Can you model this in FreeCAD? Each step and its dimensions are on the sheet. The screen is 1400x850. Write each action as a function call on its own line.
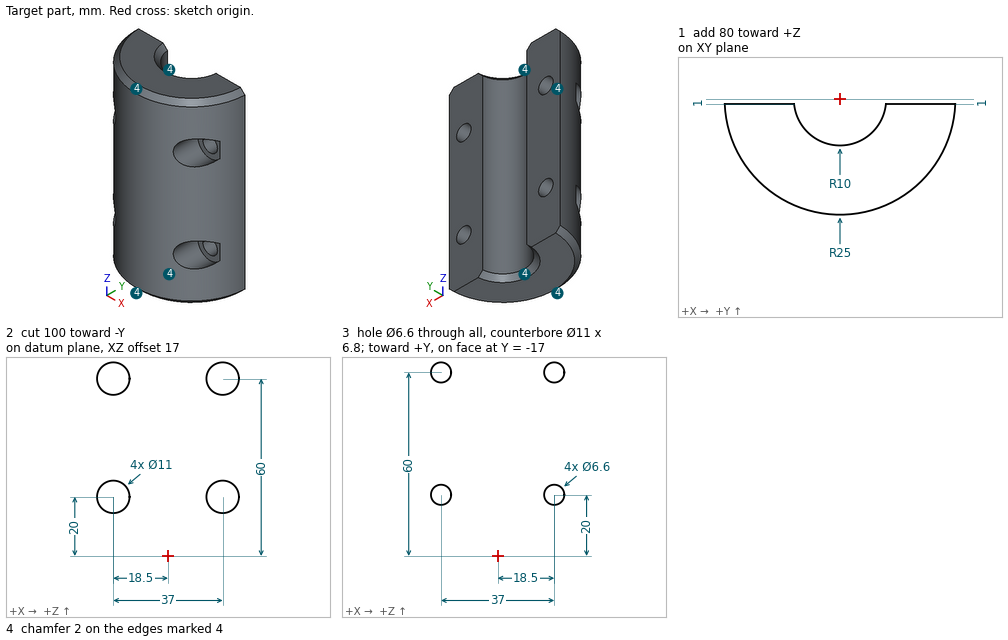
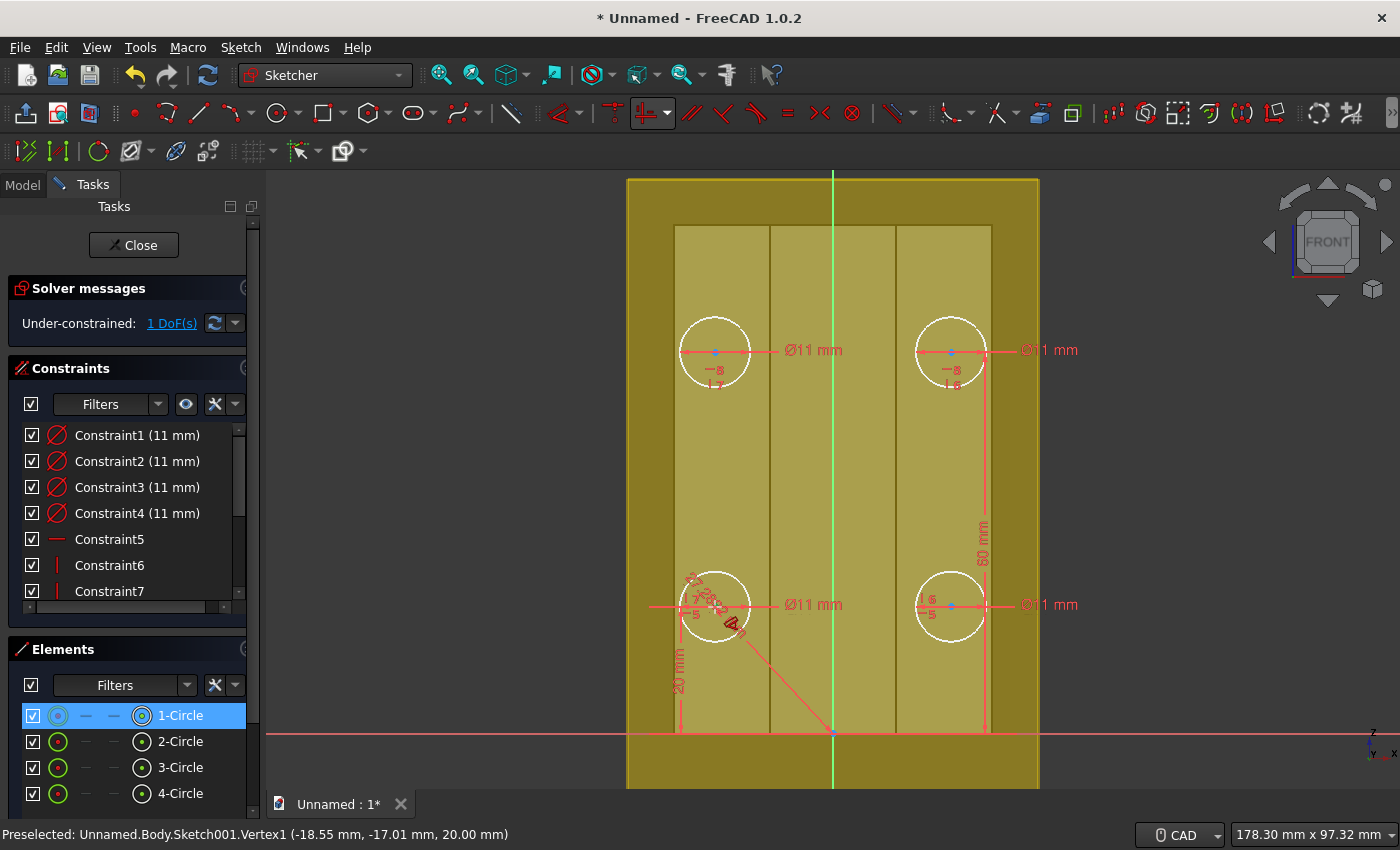
click(951, 607)
click(779, 641)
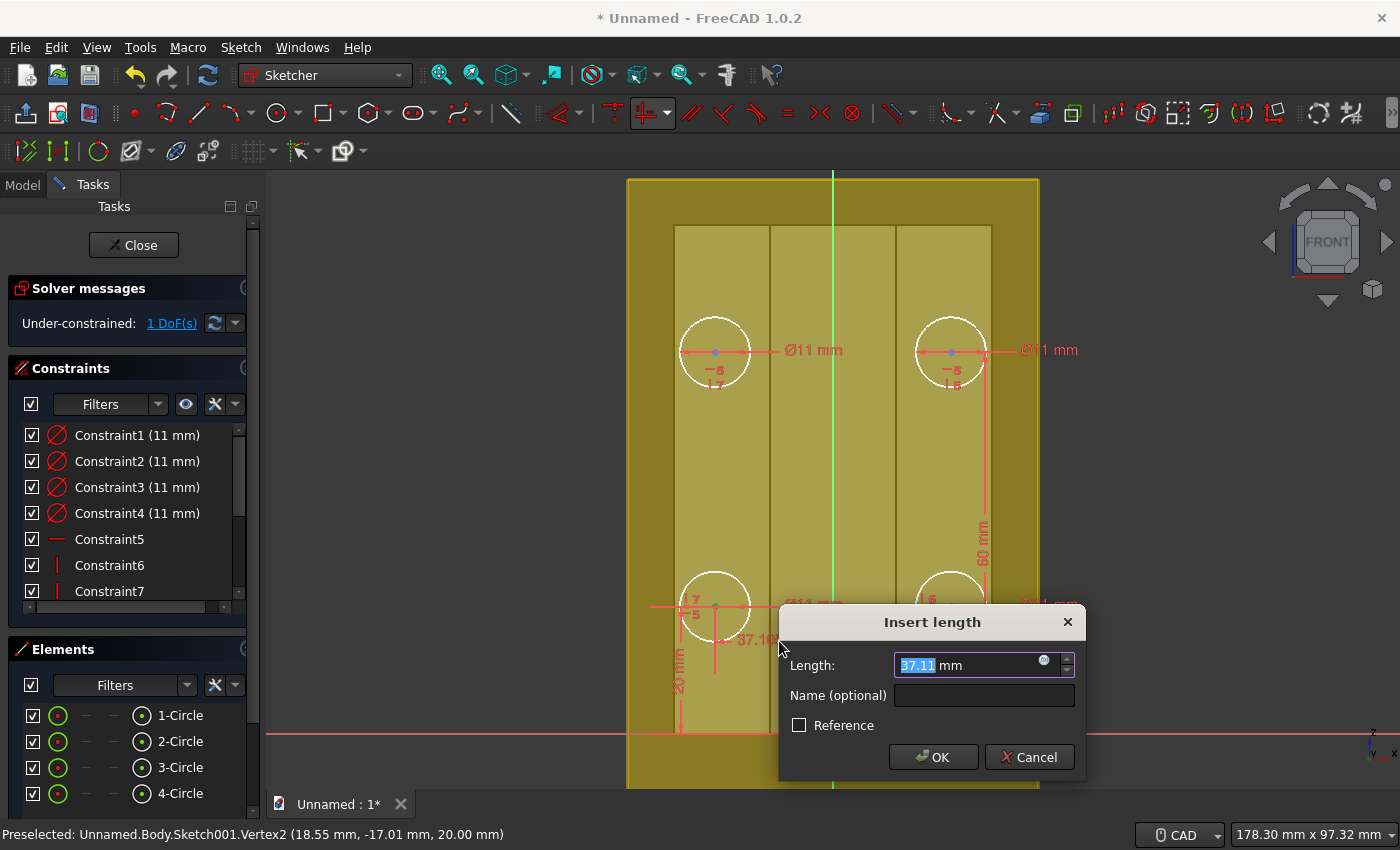
text(37)
key(Return)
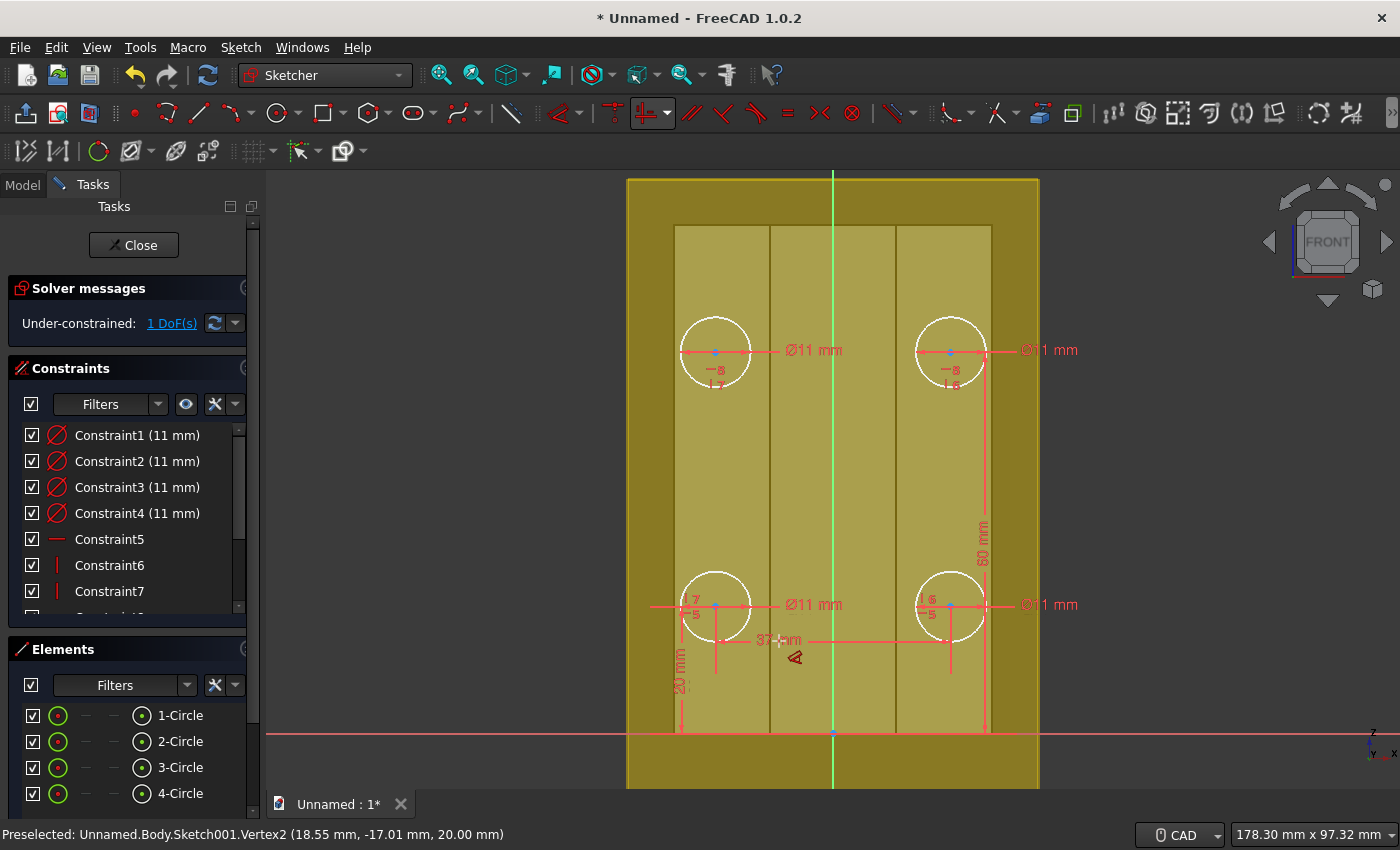
click(716, 607)
click(774, 573)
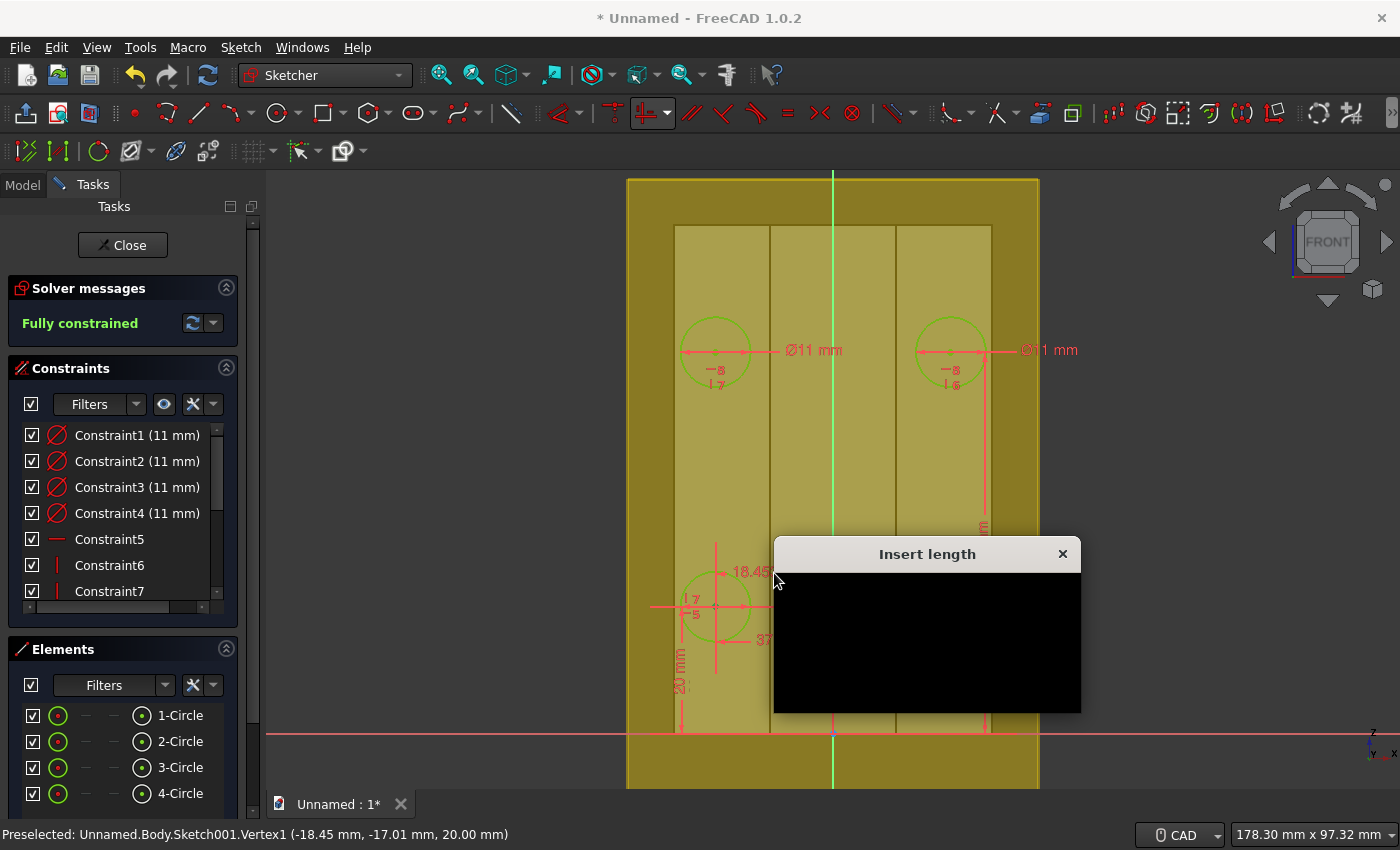
text(18.5)
key(Return)
key(Escape)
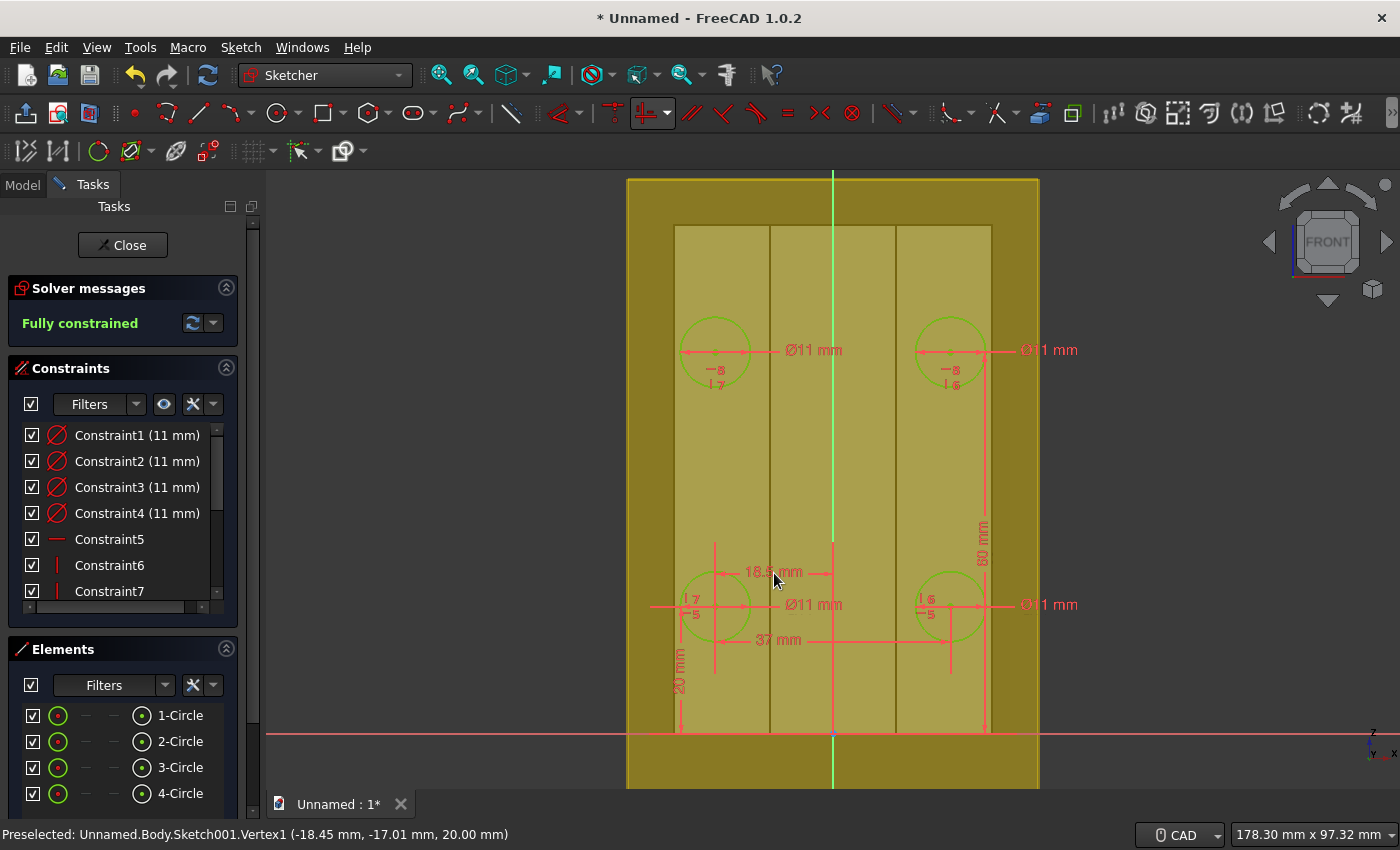
click(123, 245)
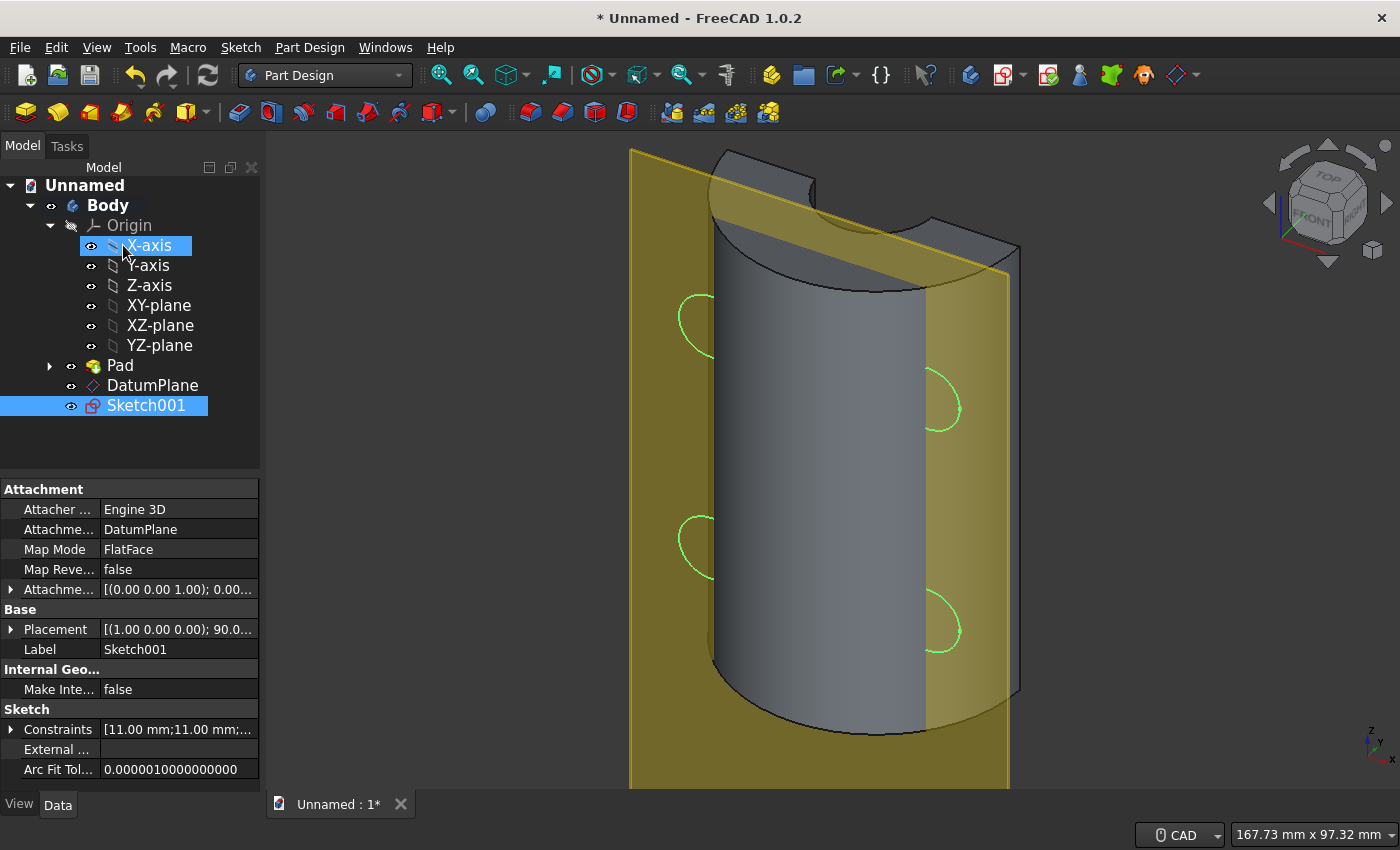
click(240, 112)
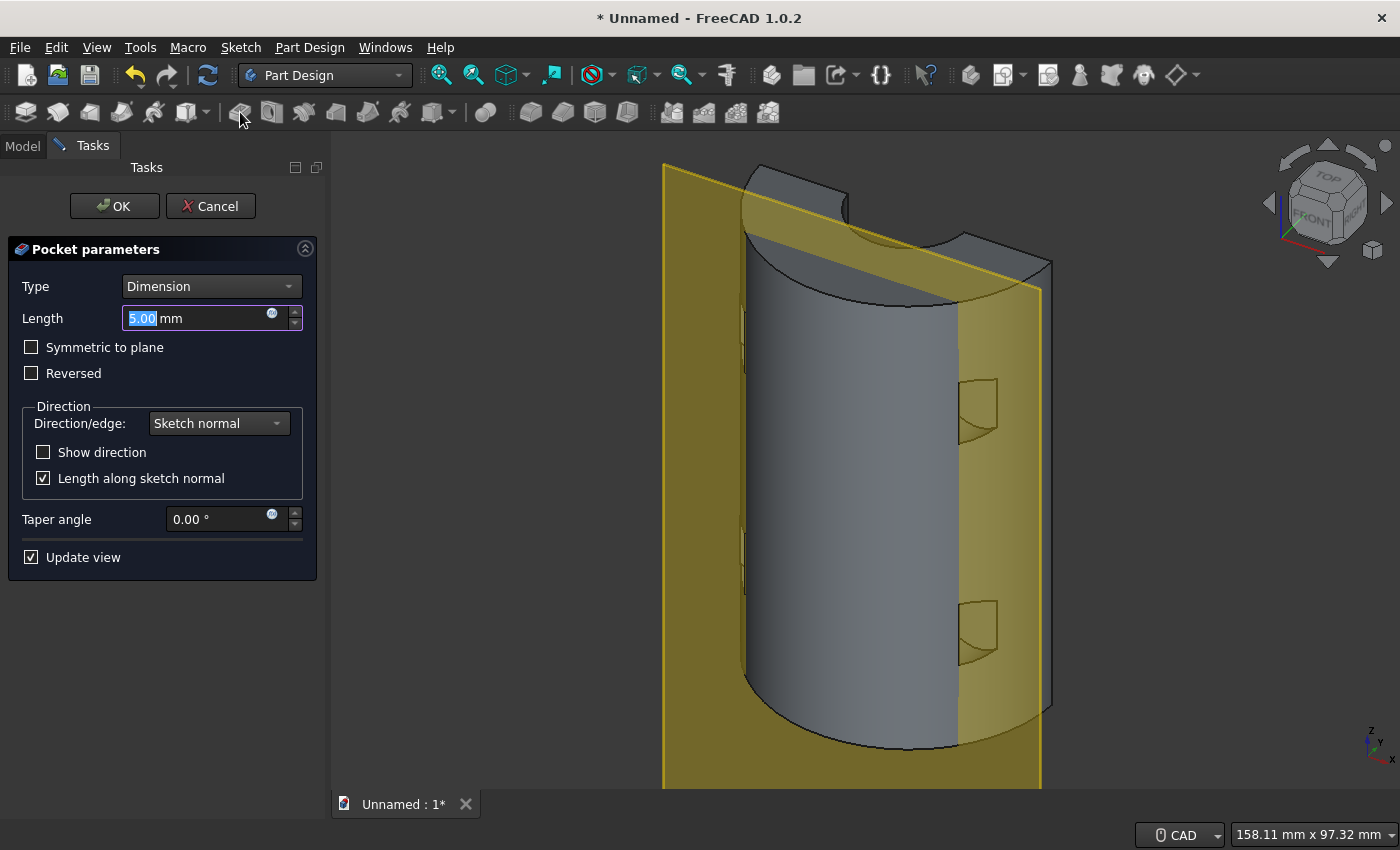
text(100)
key(Tab)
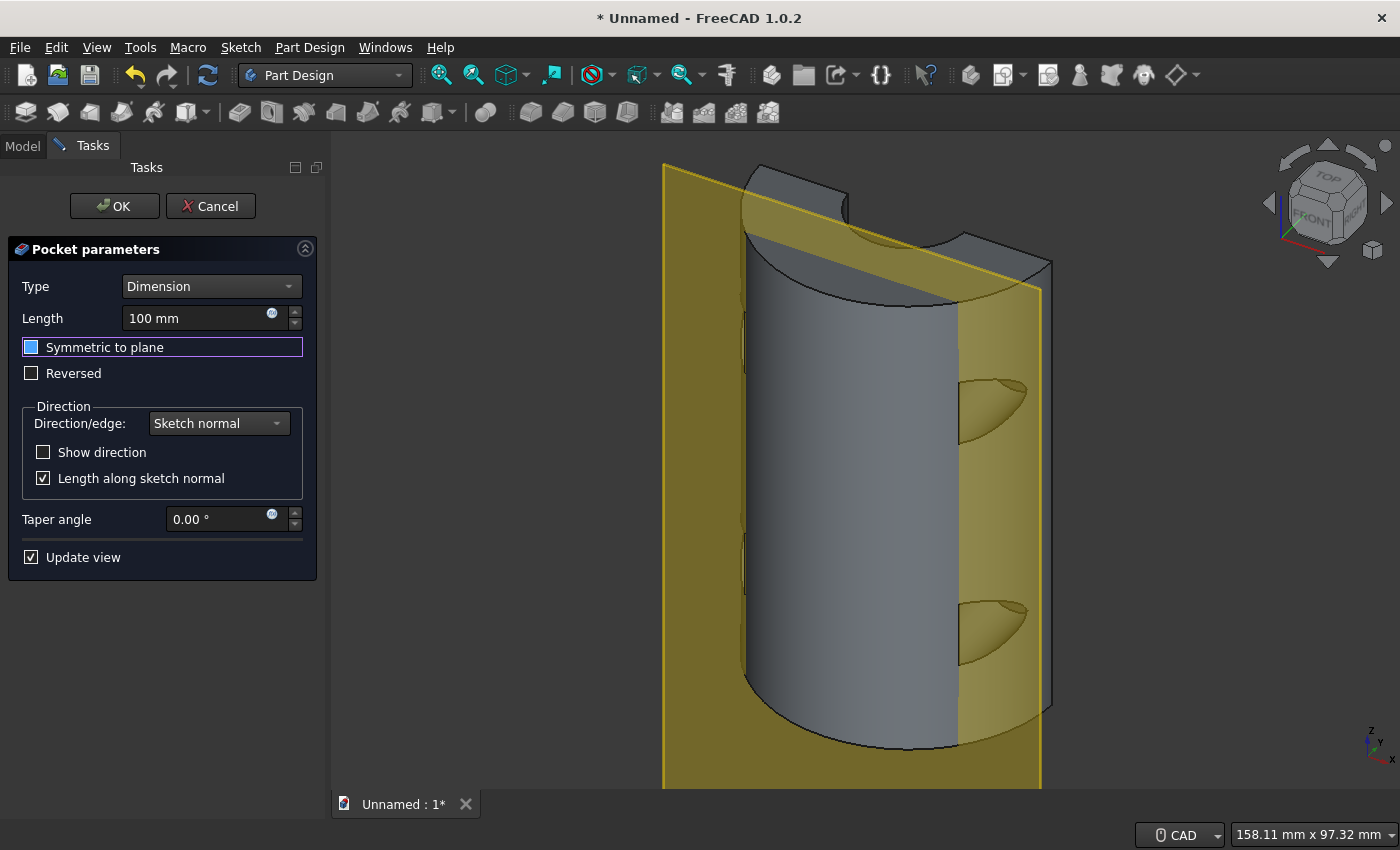
click(30, 373)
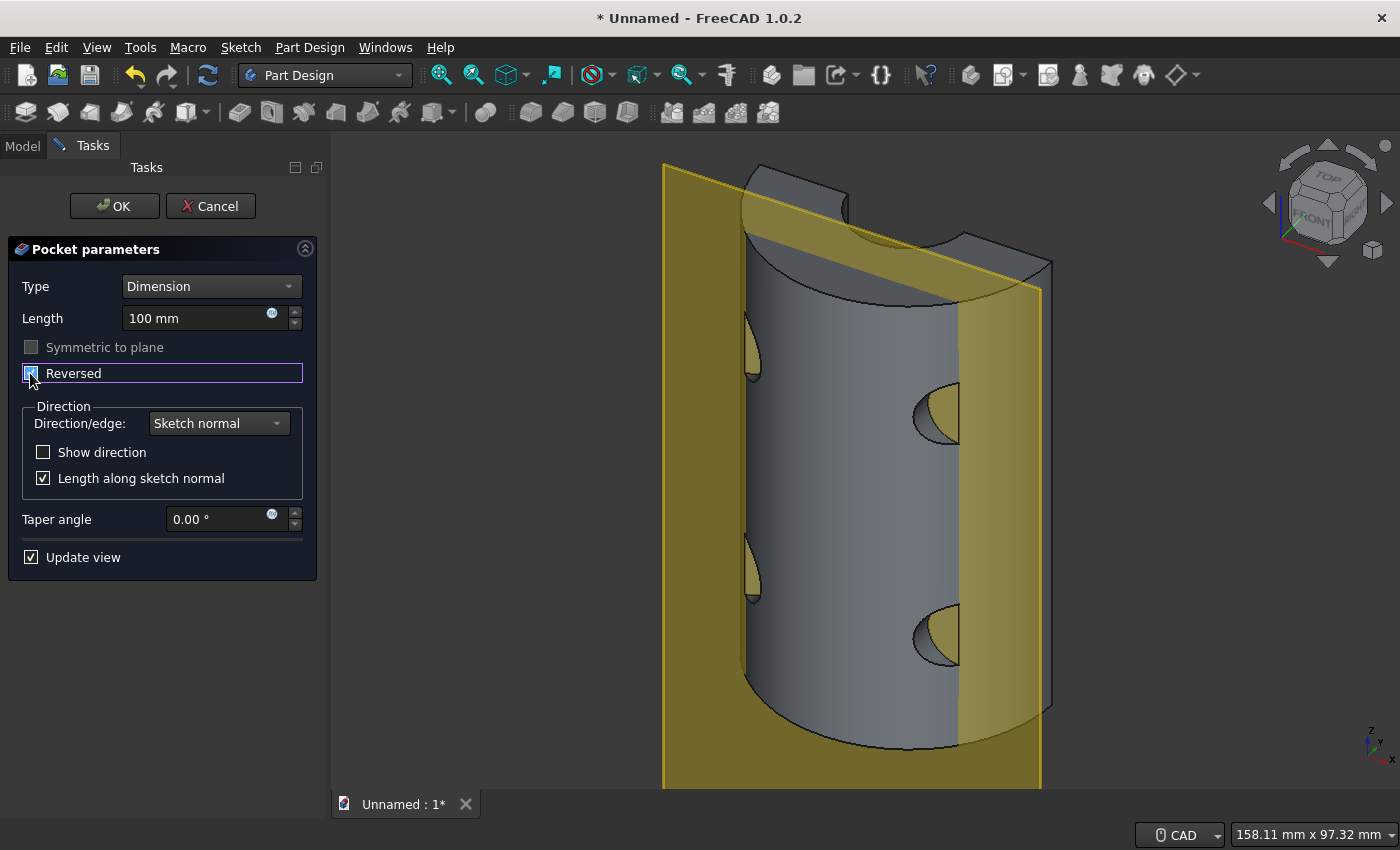
click(115, 206)